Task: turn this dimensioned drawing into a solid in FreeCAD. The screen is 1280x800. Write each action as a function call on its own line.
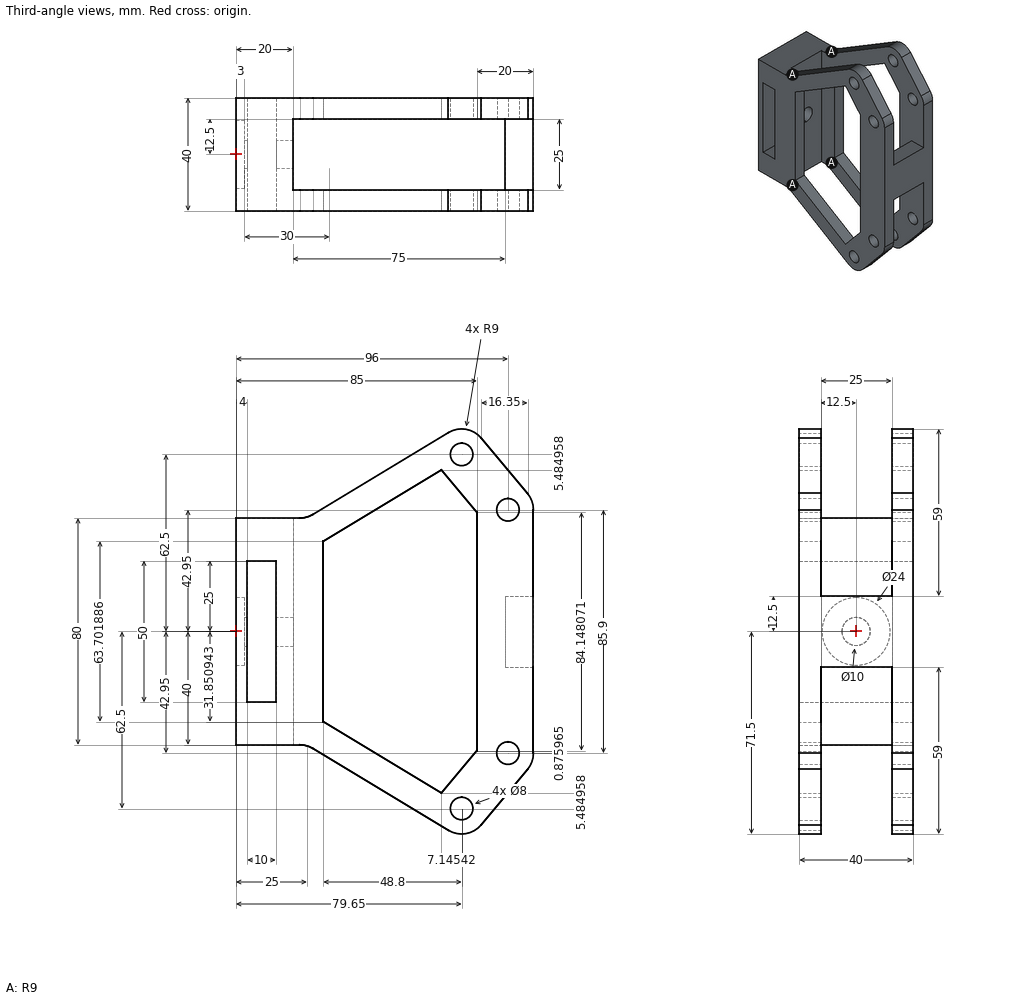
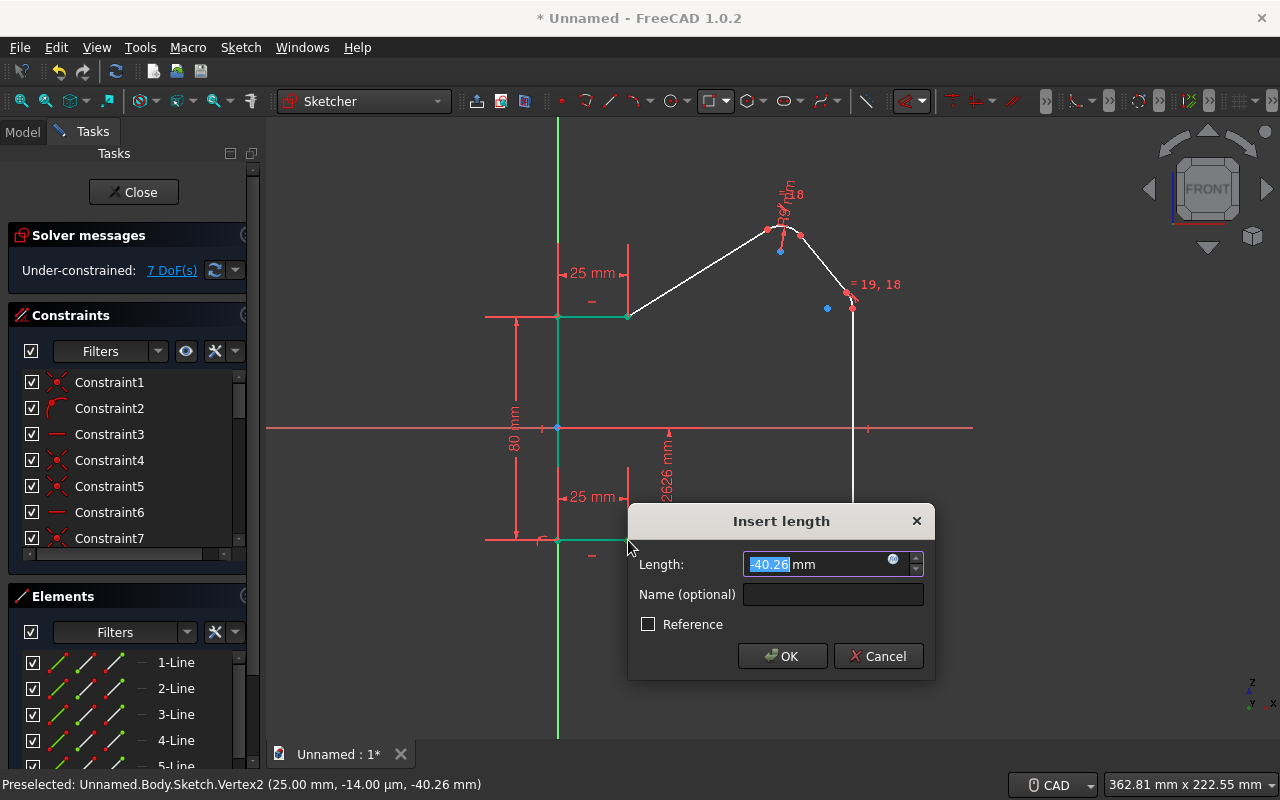
text(-40)
key(Return)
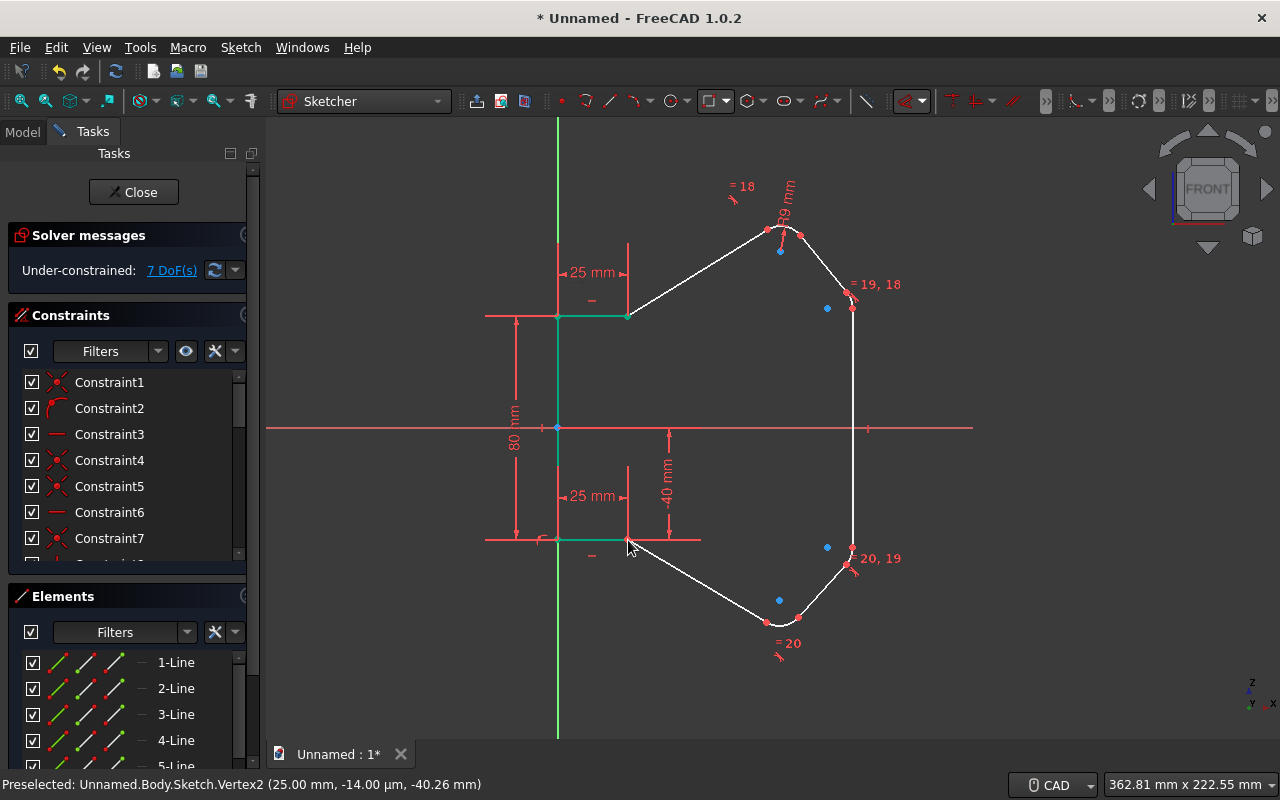
click(827, 308)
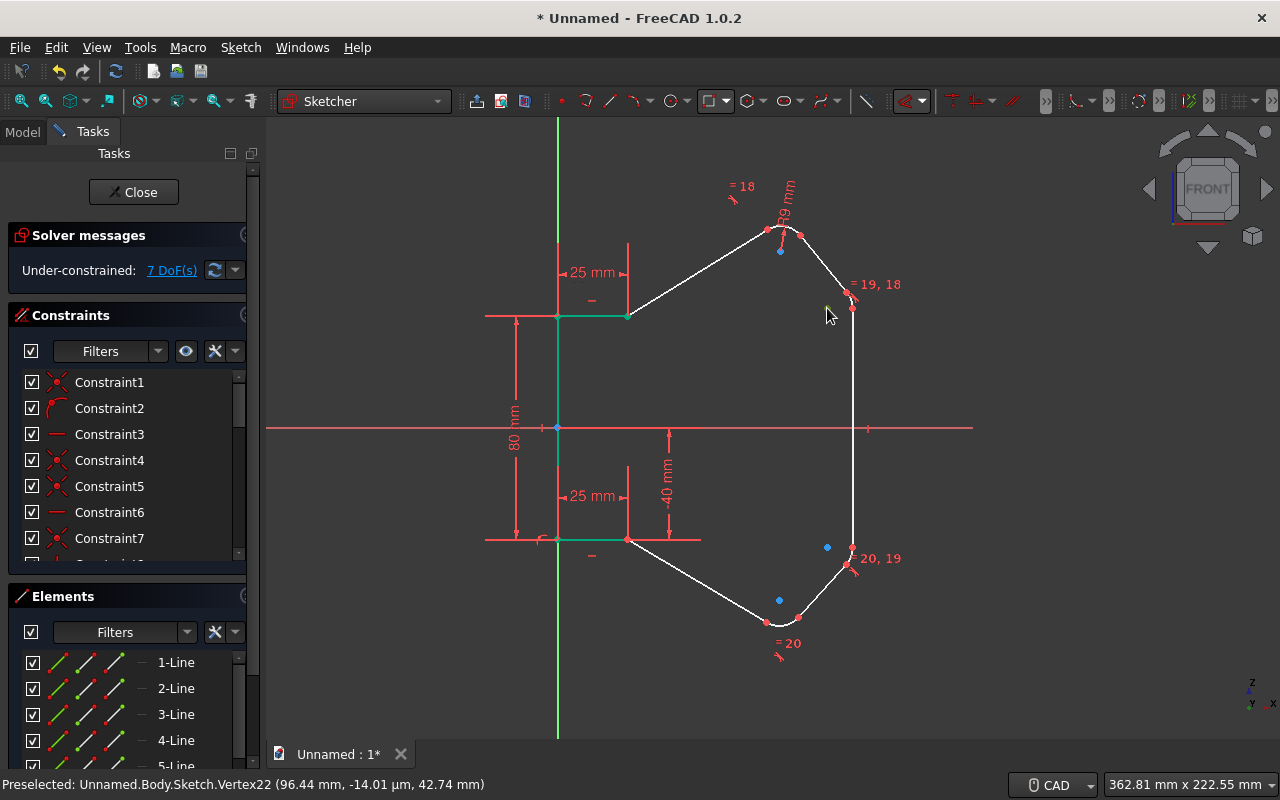
key(l)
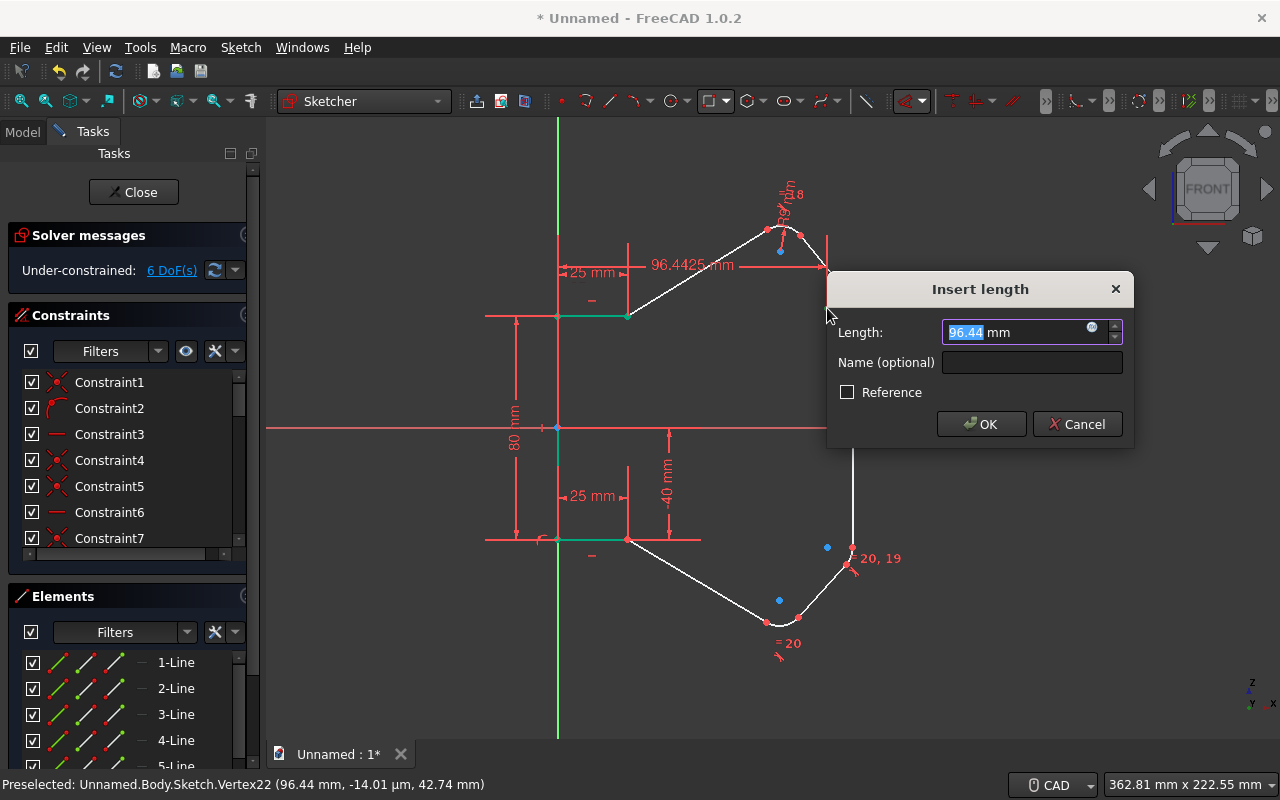
text(96)
key(Return)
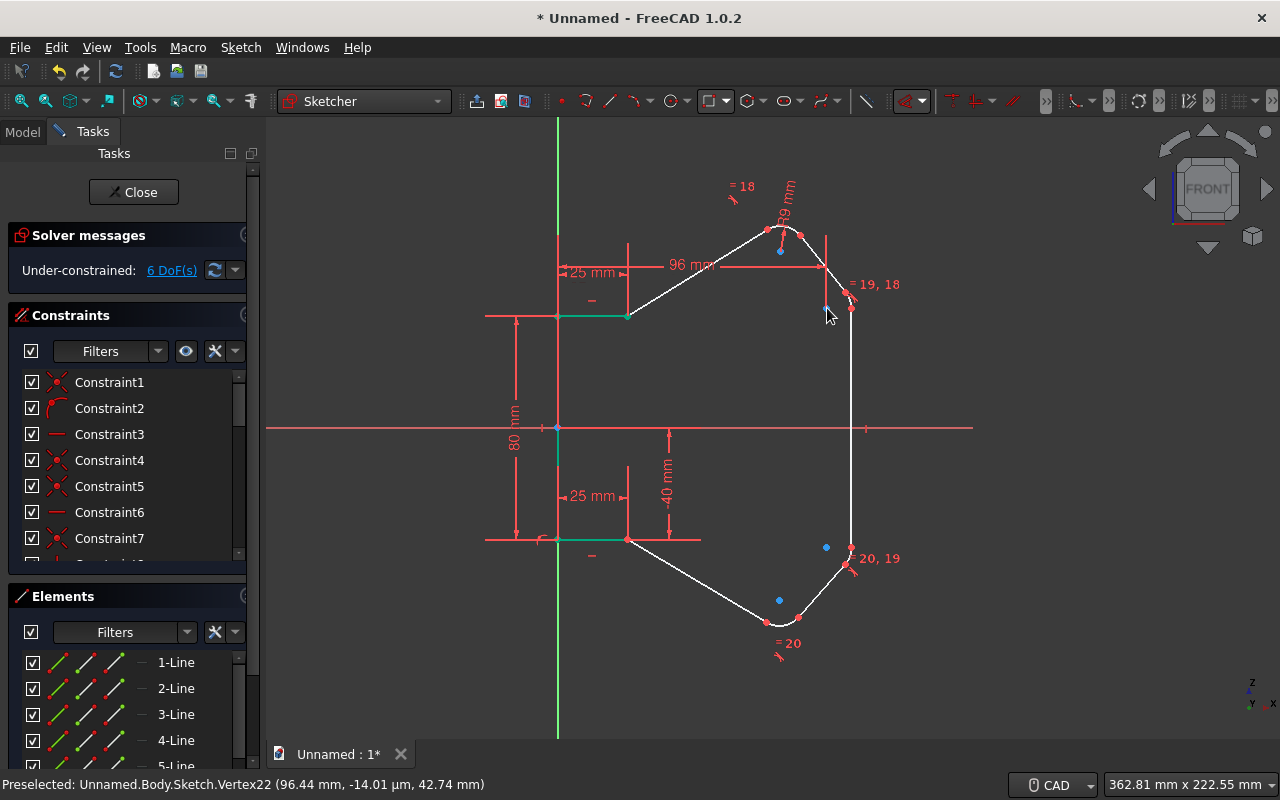
click(851, 380)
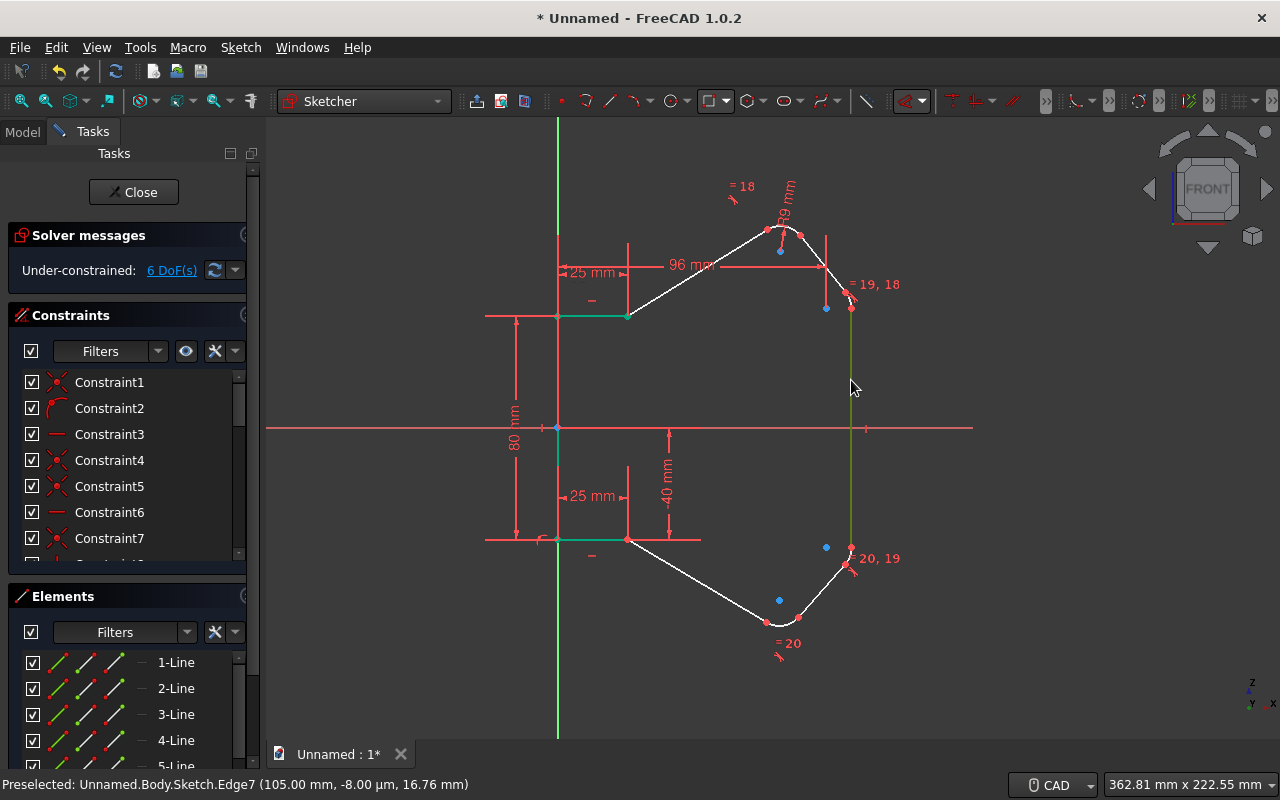
key(i)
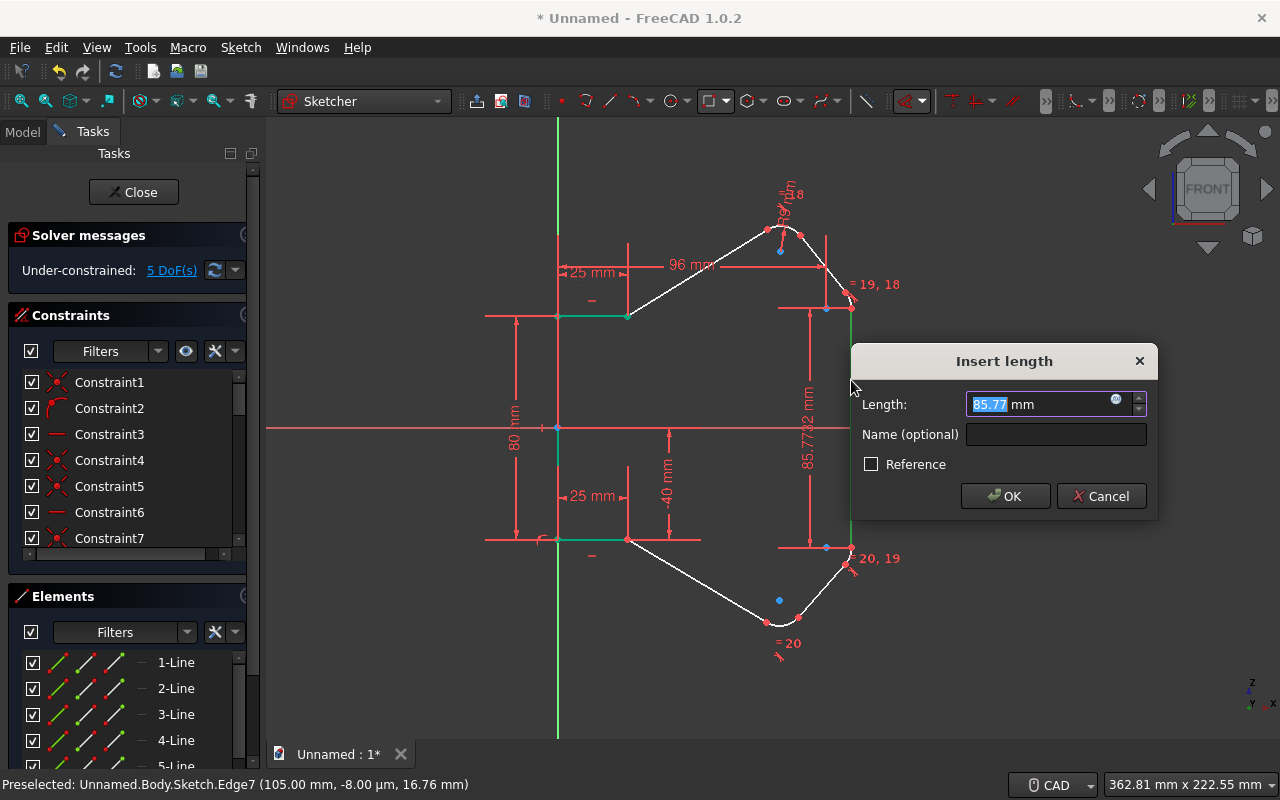
text(85.9)
key(Return)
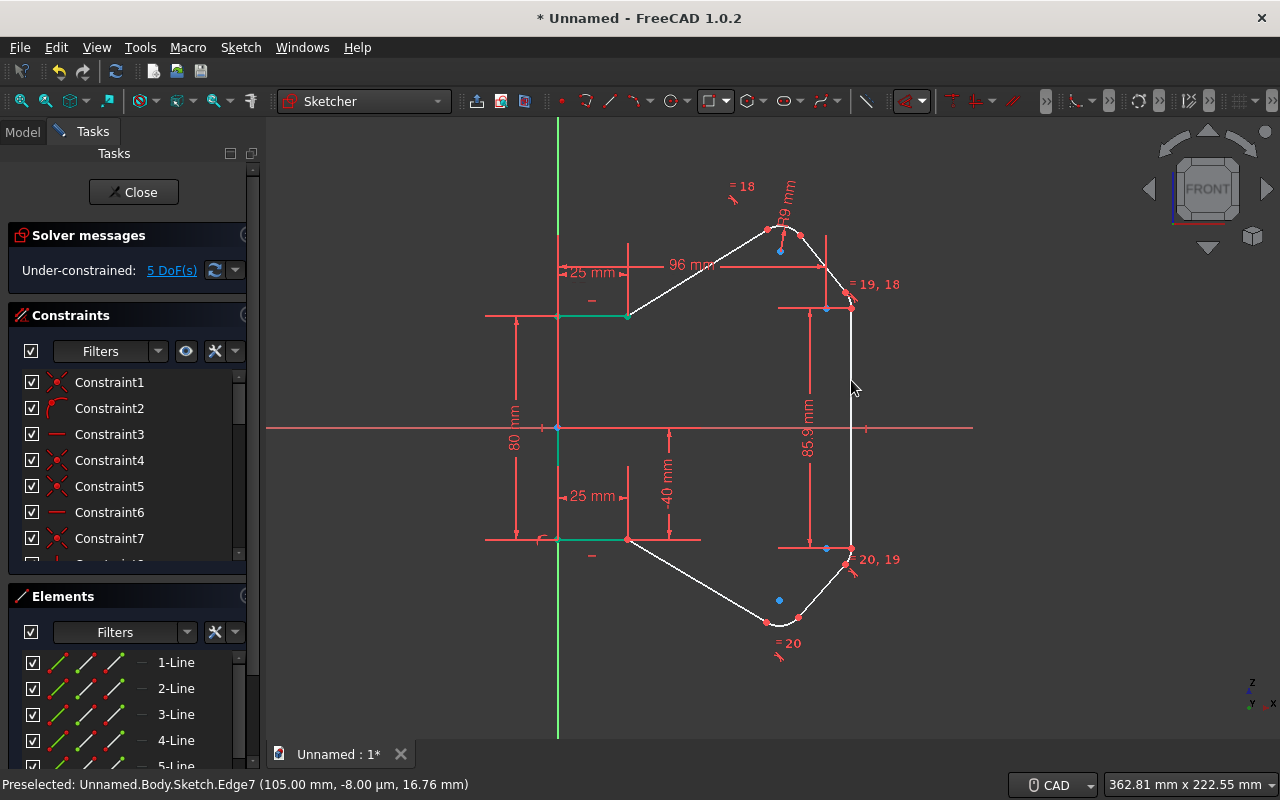
click(781, 251)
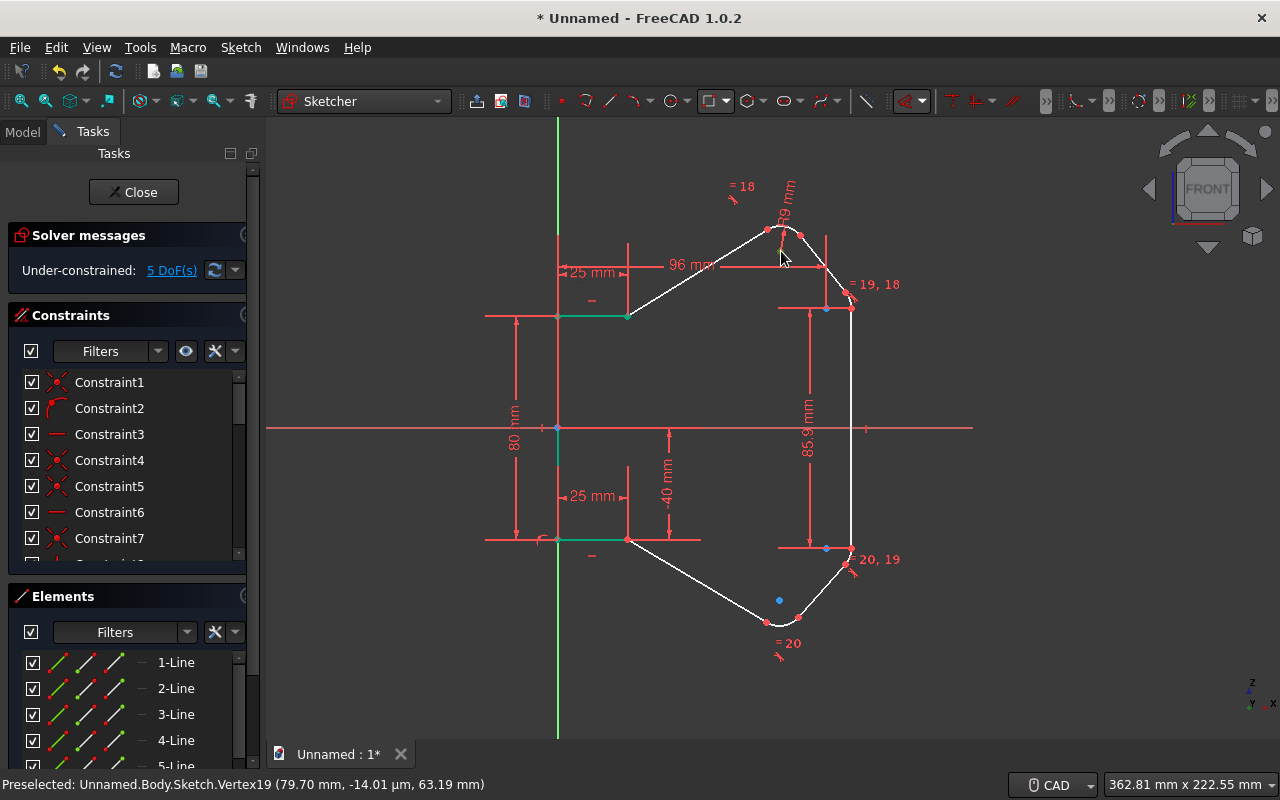
key(i)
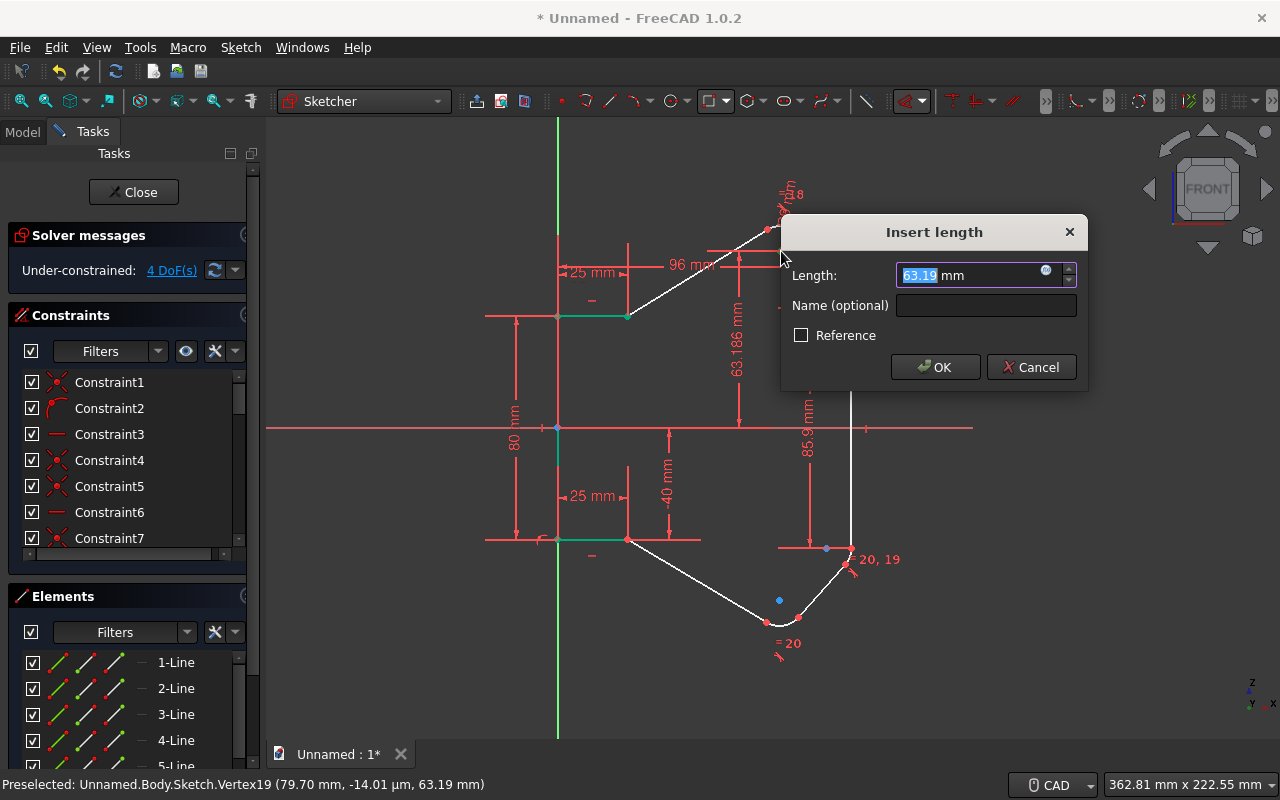
text(62.5)
key(Return)